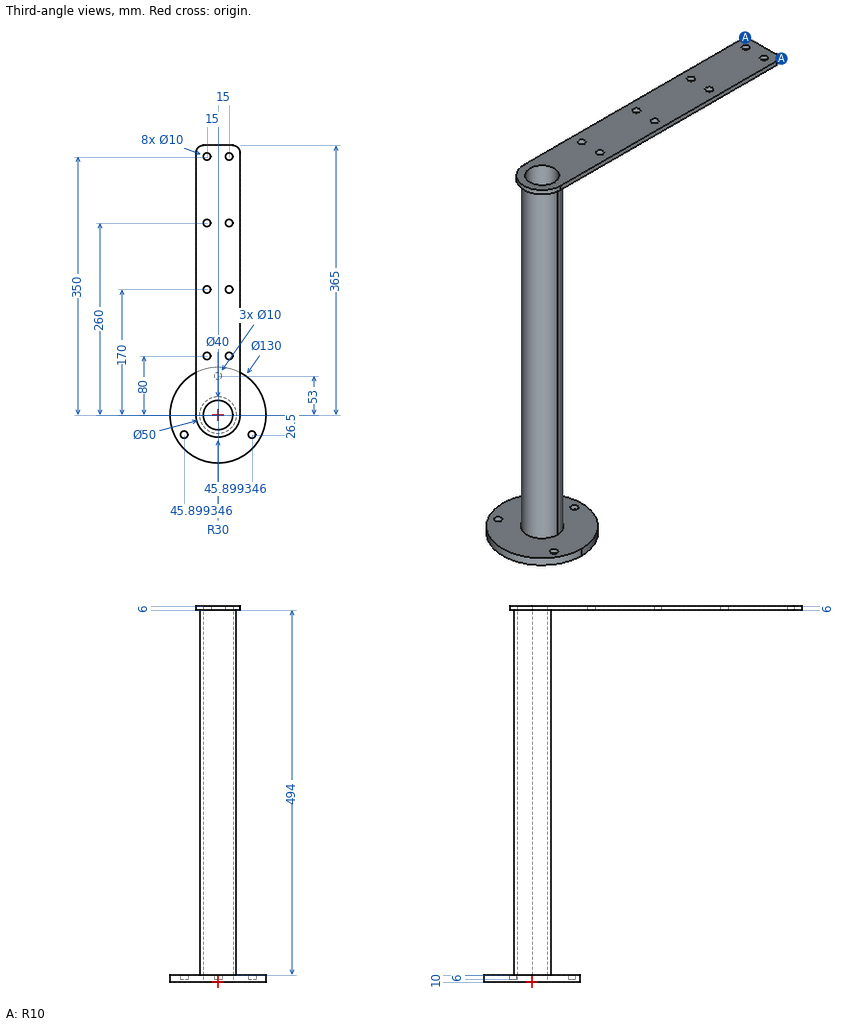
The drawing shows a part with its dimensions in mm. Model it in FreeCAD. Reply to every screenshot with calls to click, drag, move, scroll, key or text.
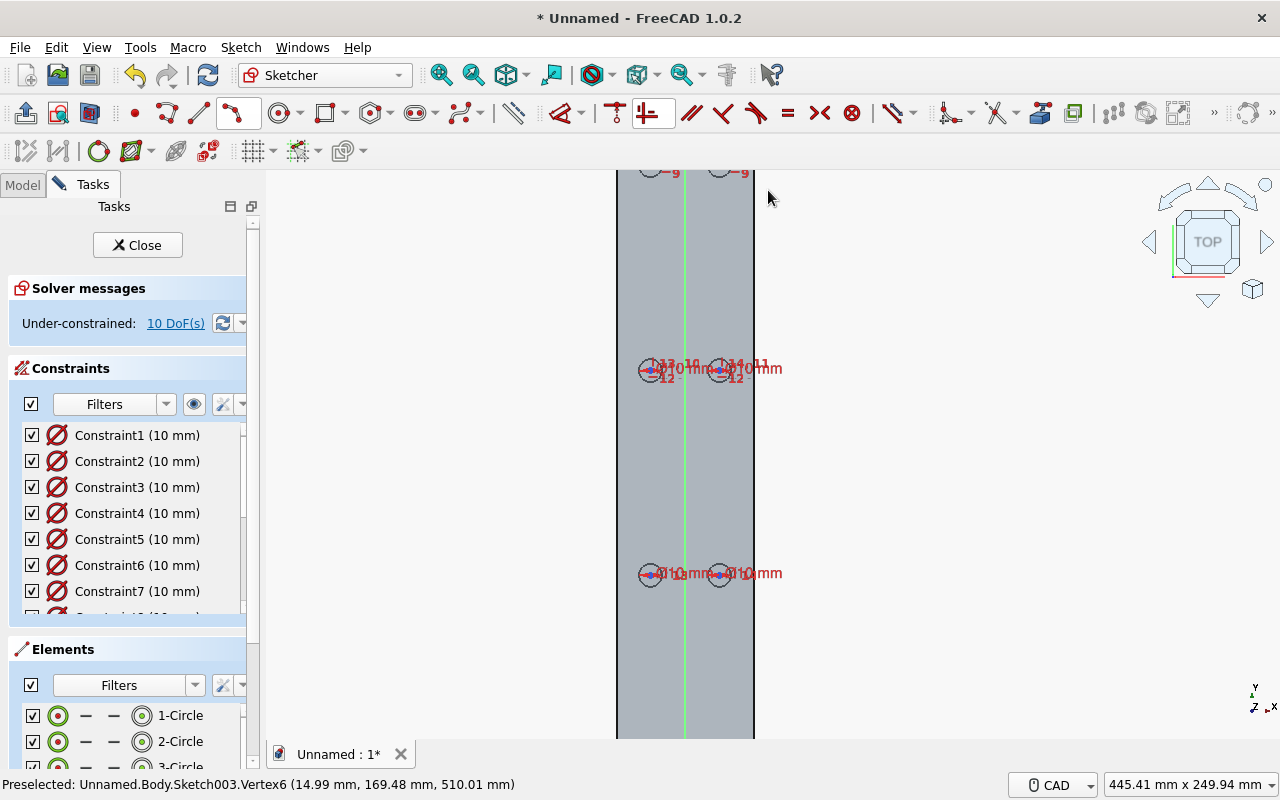
click(650, 575)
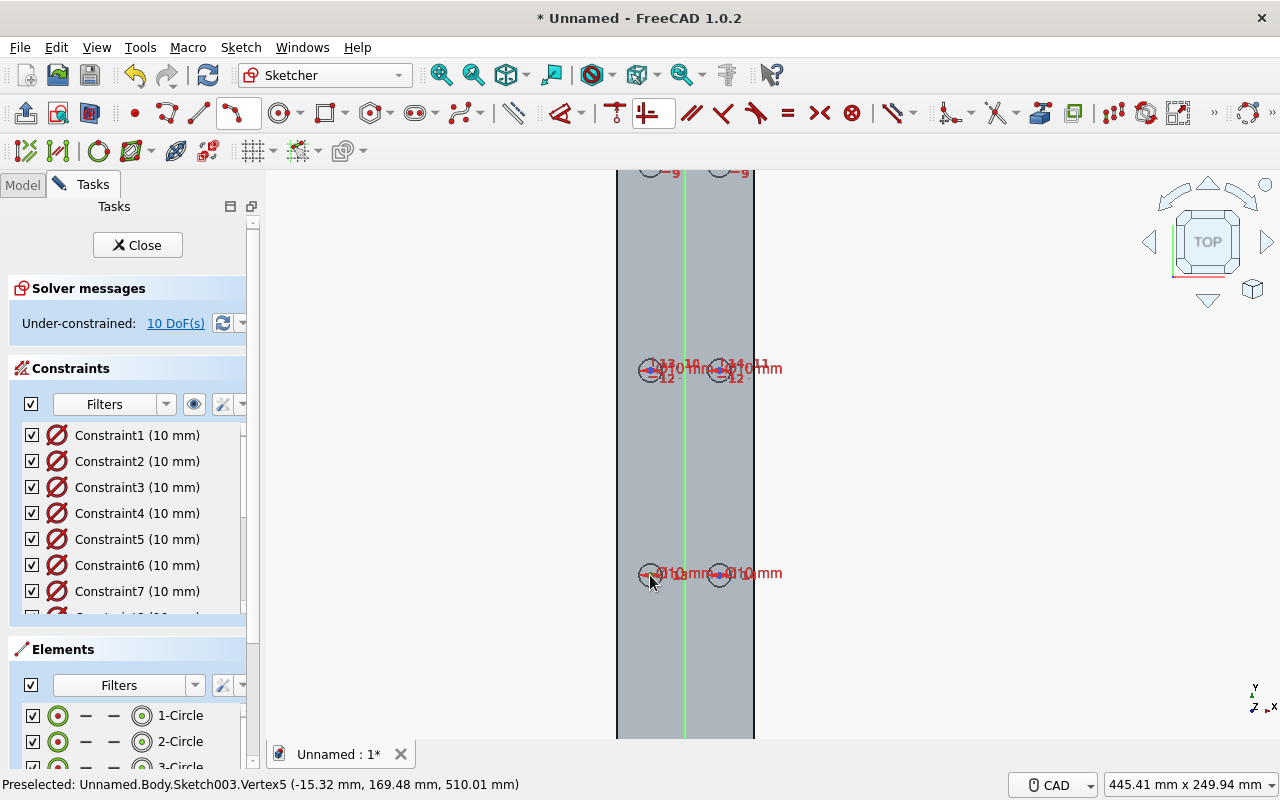
click(719, 575)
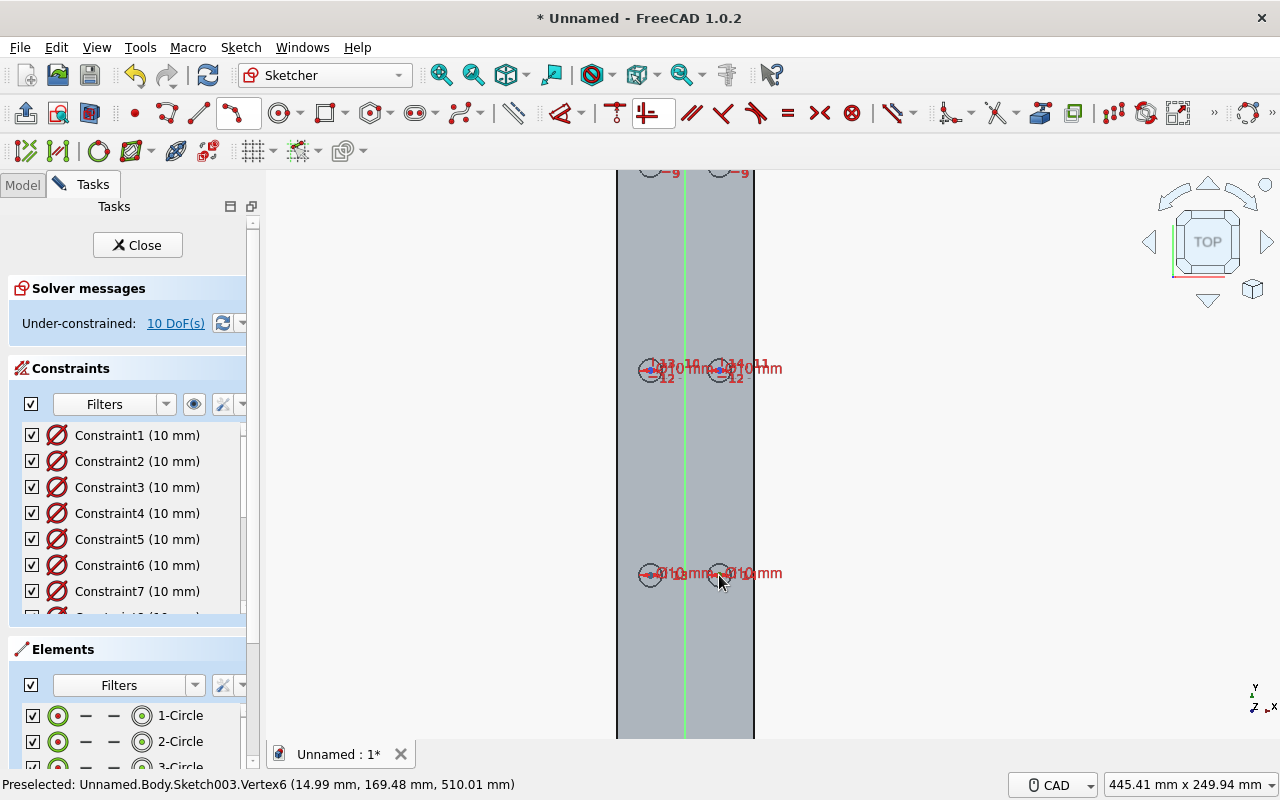
key(h)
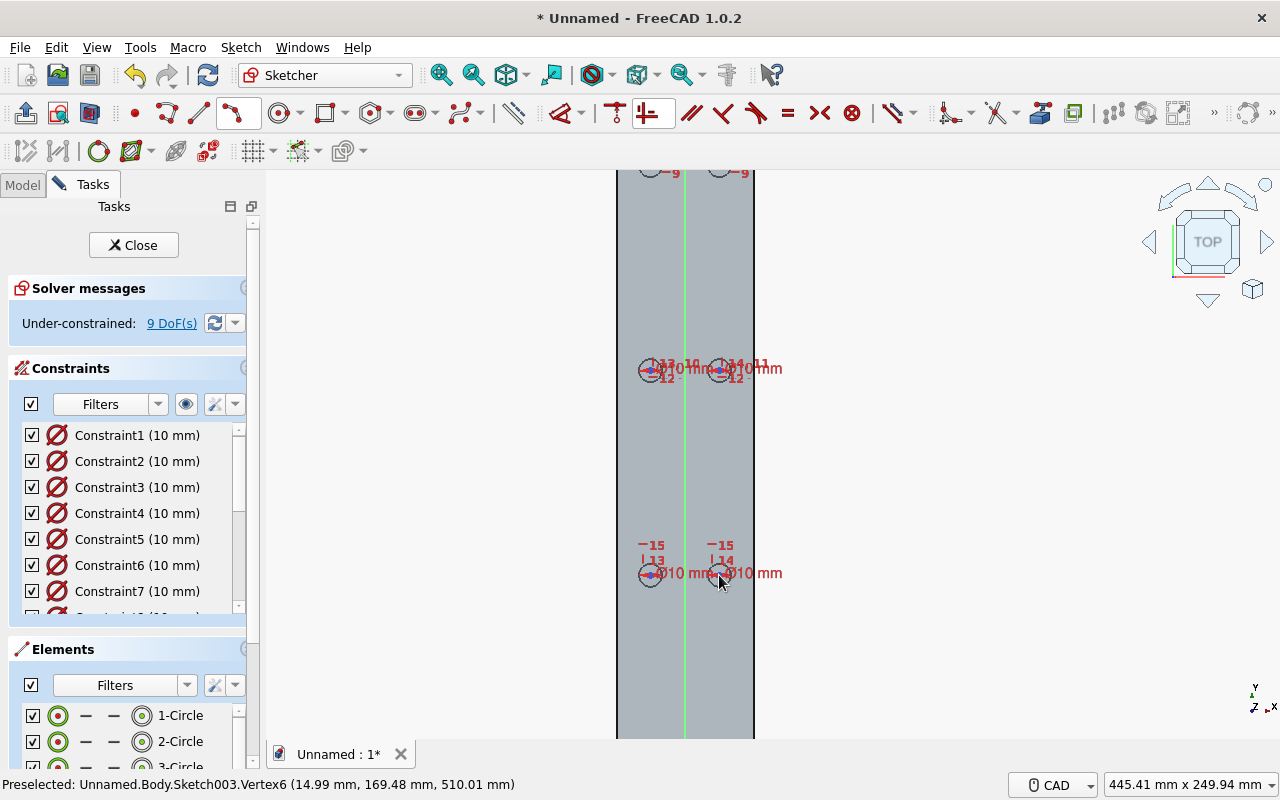
click(650, 575)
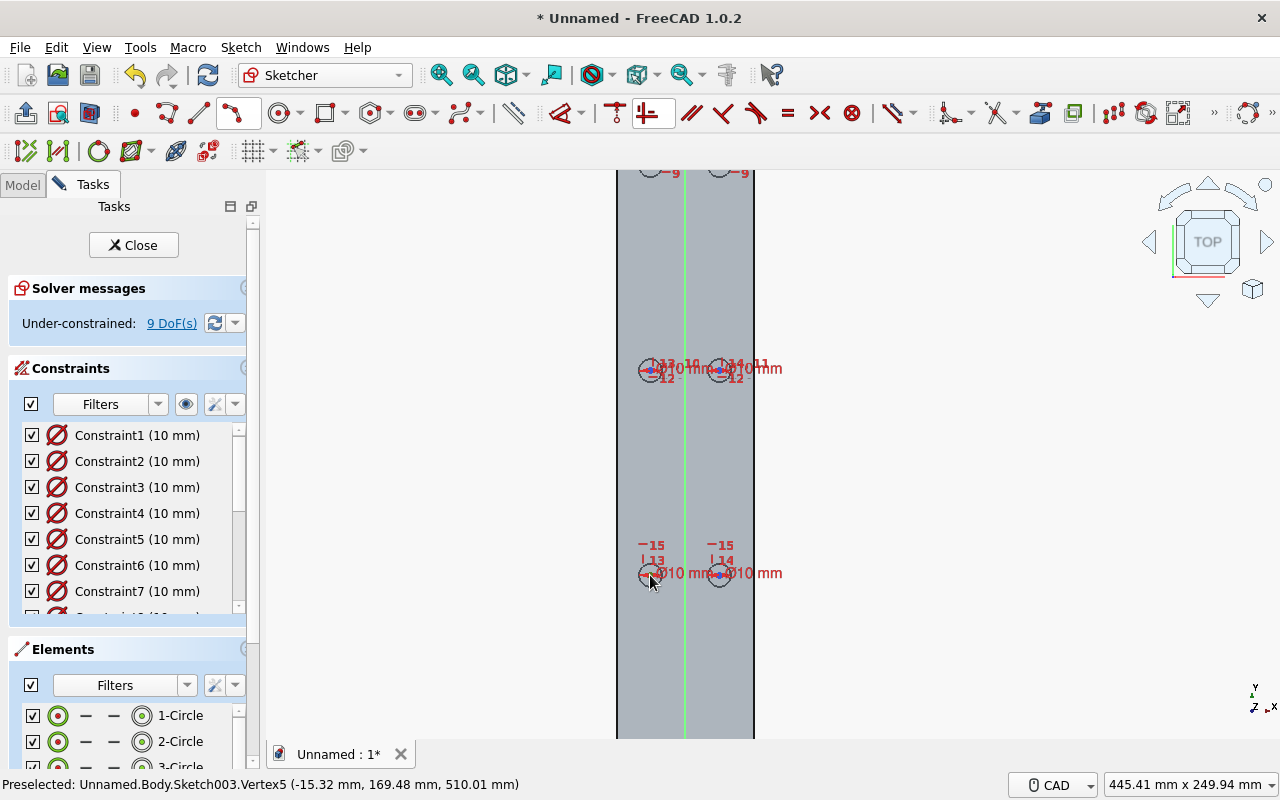
scroll(720, 371, down, 4)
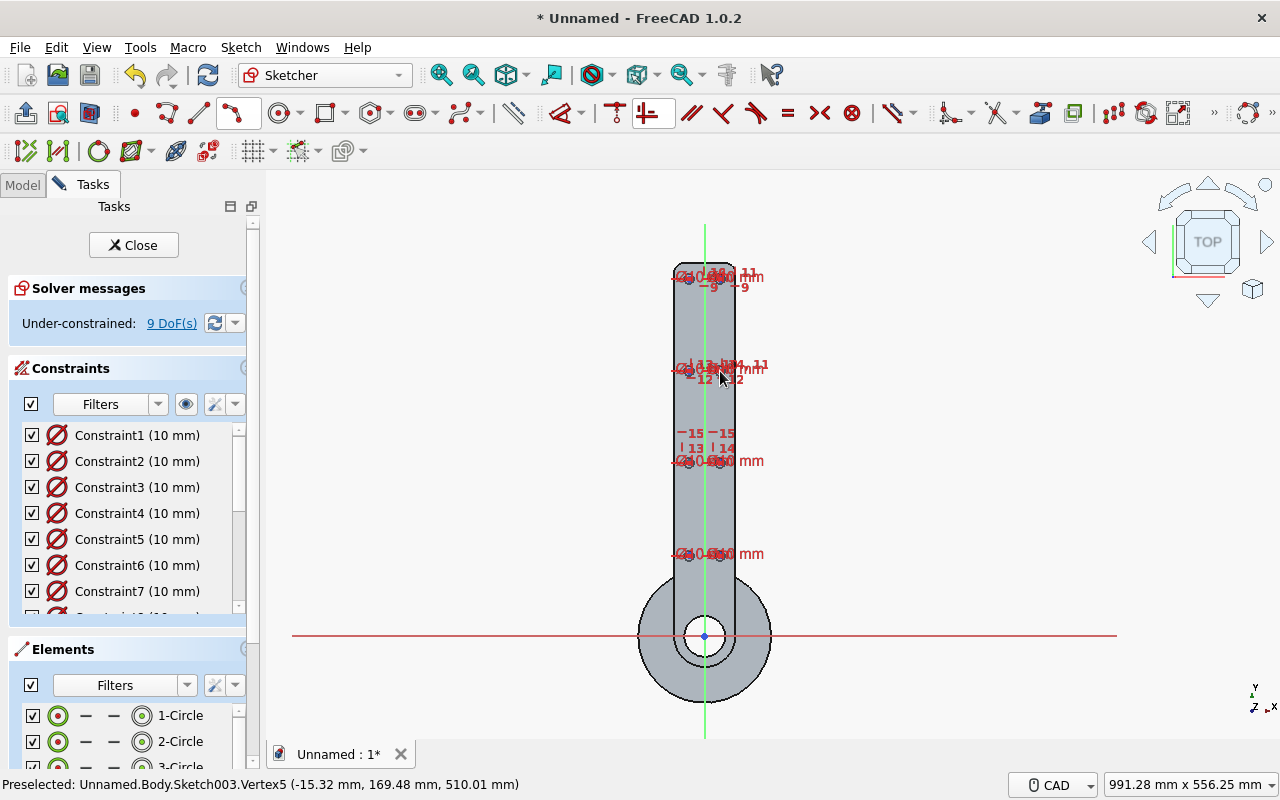
click(689, 556)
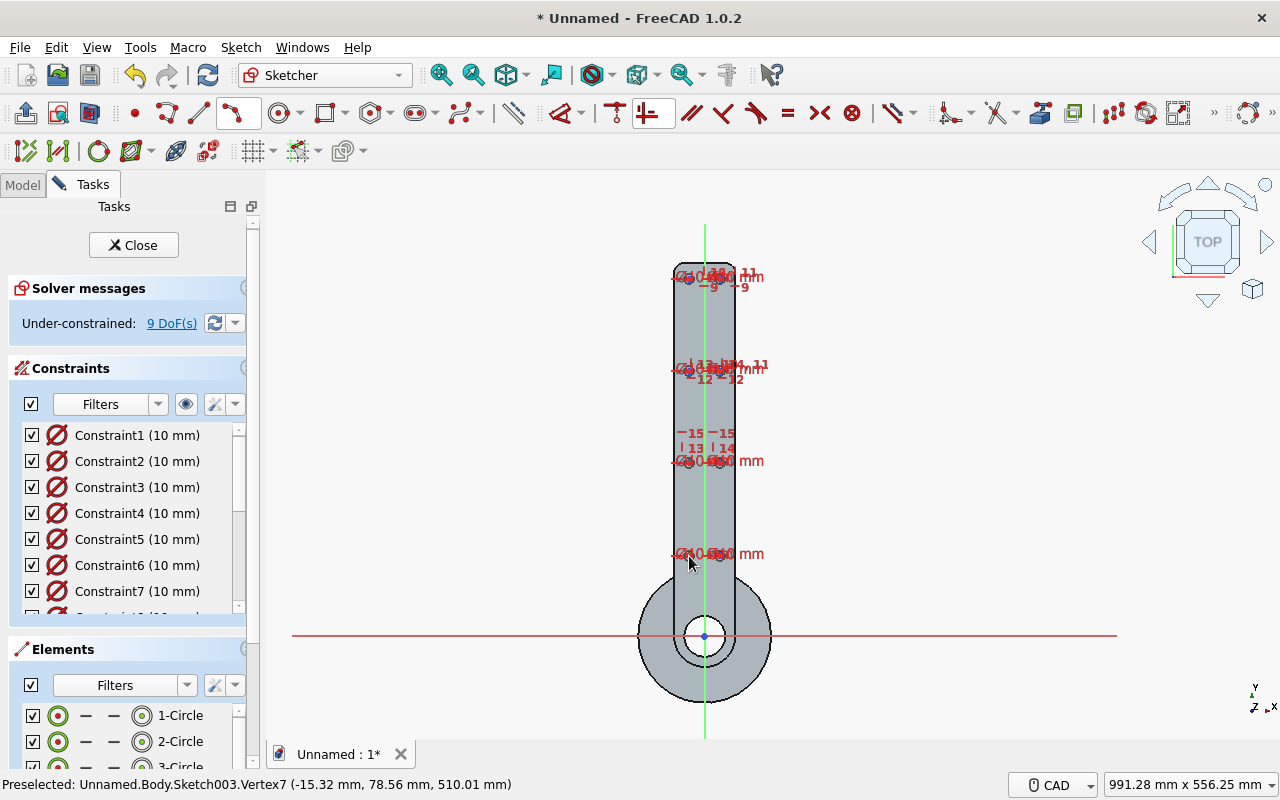
click(670, 114)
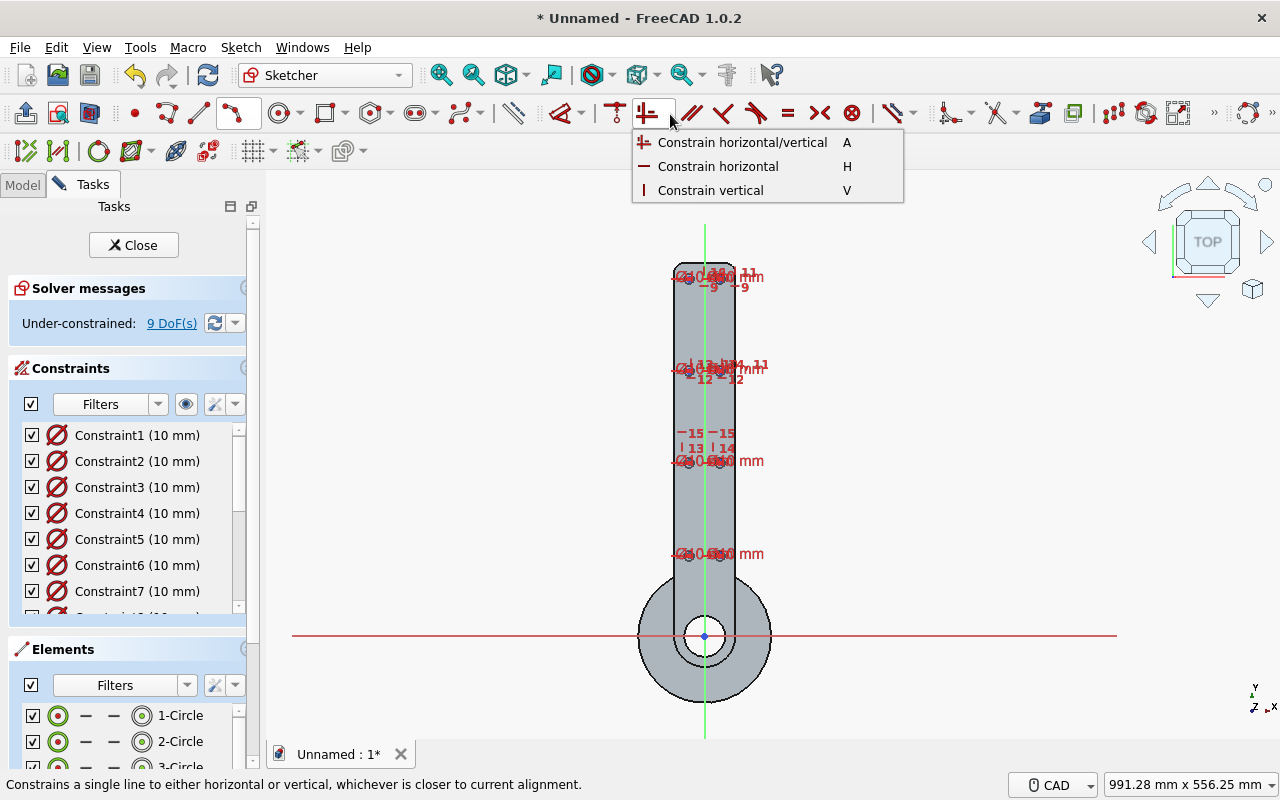
click(768, 190)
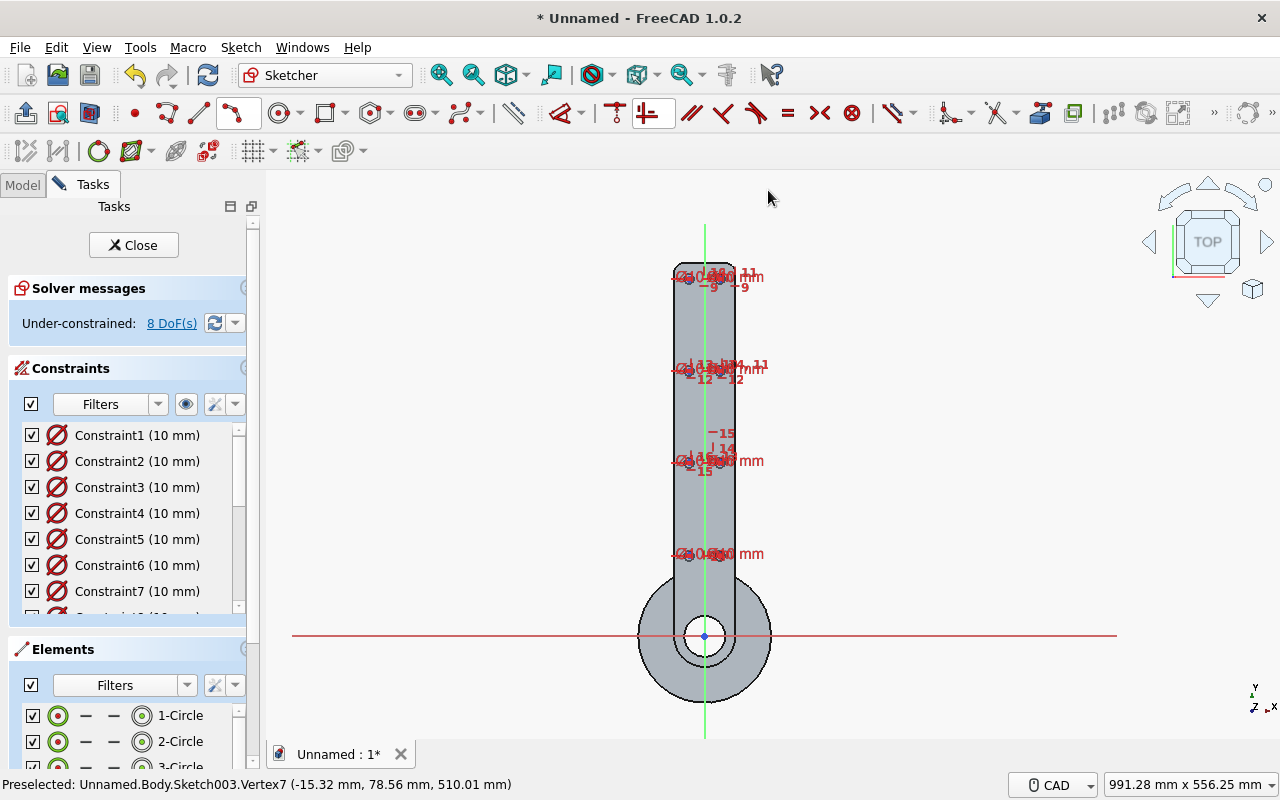
click(720, 463)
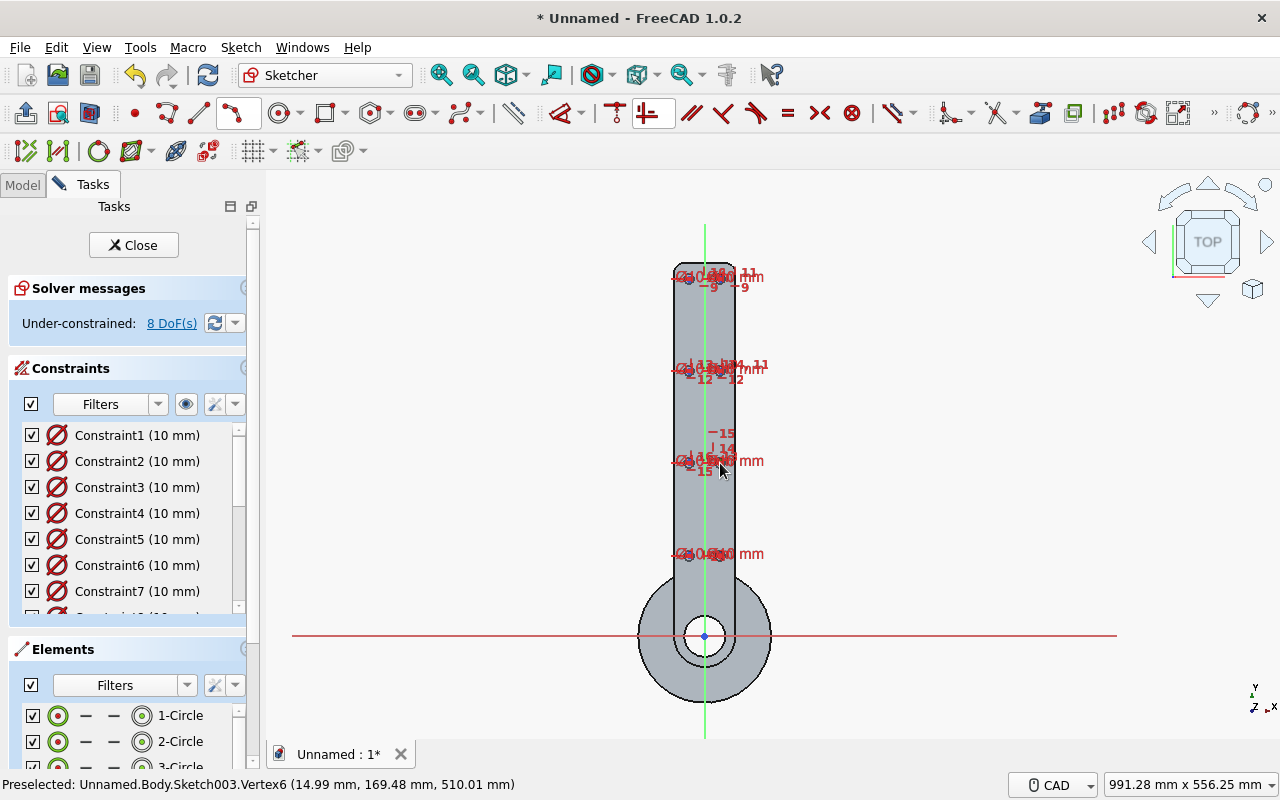
scroll(720, 556, up, 4)